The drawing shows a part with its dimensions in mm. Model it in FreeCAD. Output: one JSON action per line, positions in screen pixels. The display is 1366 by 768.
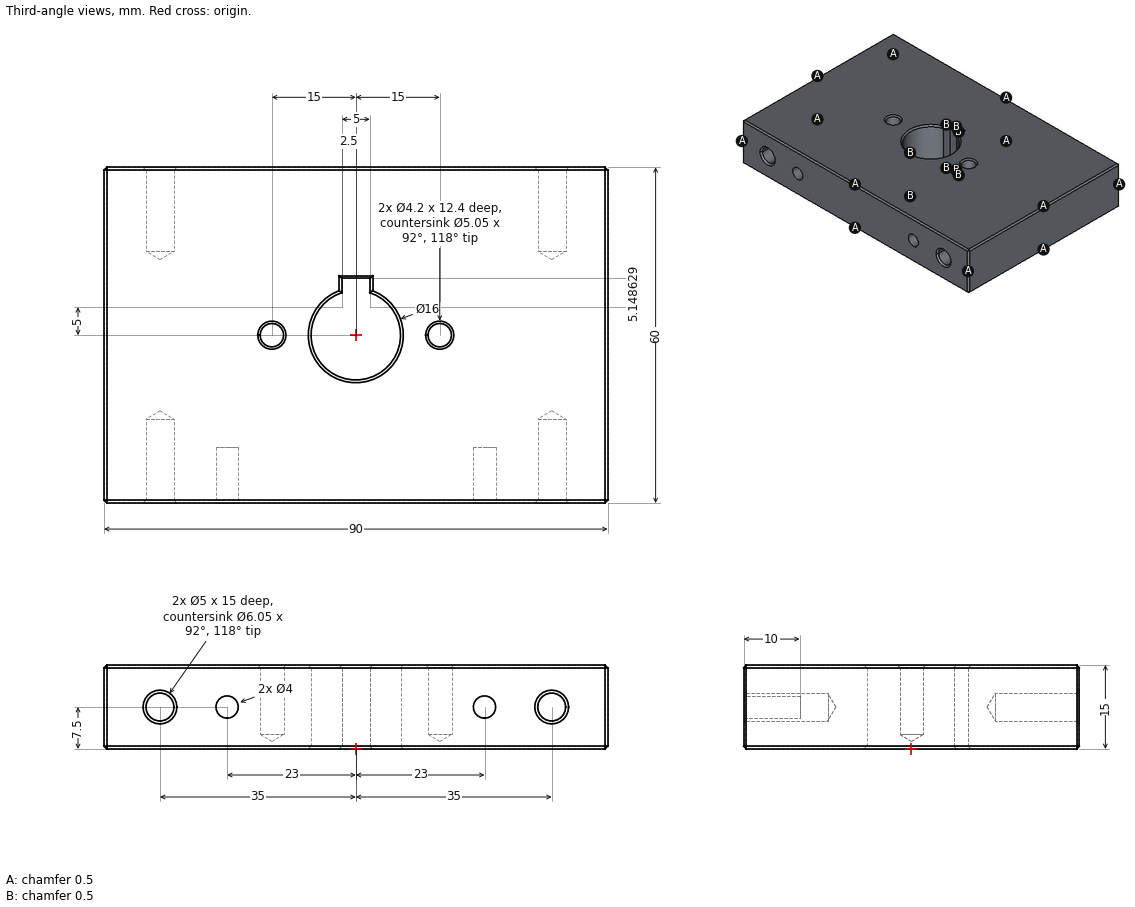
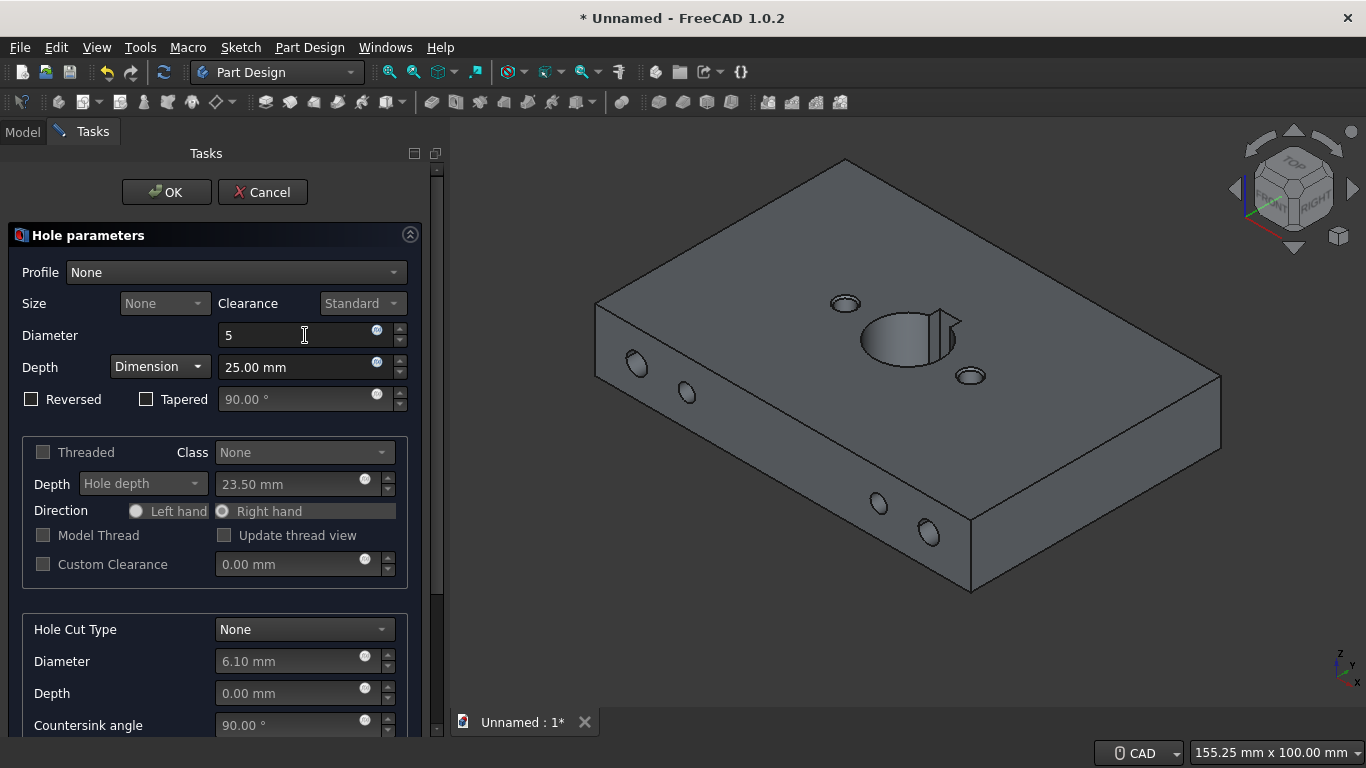
{"action": "triple_click", "coordinate": [305, 367]}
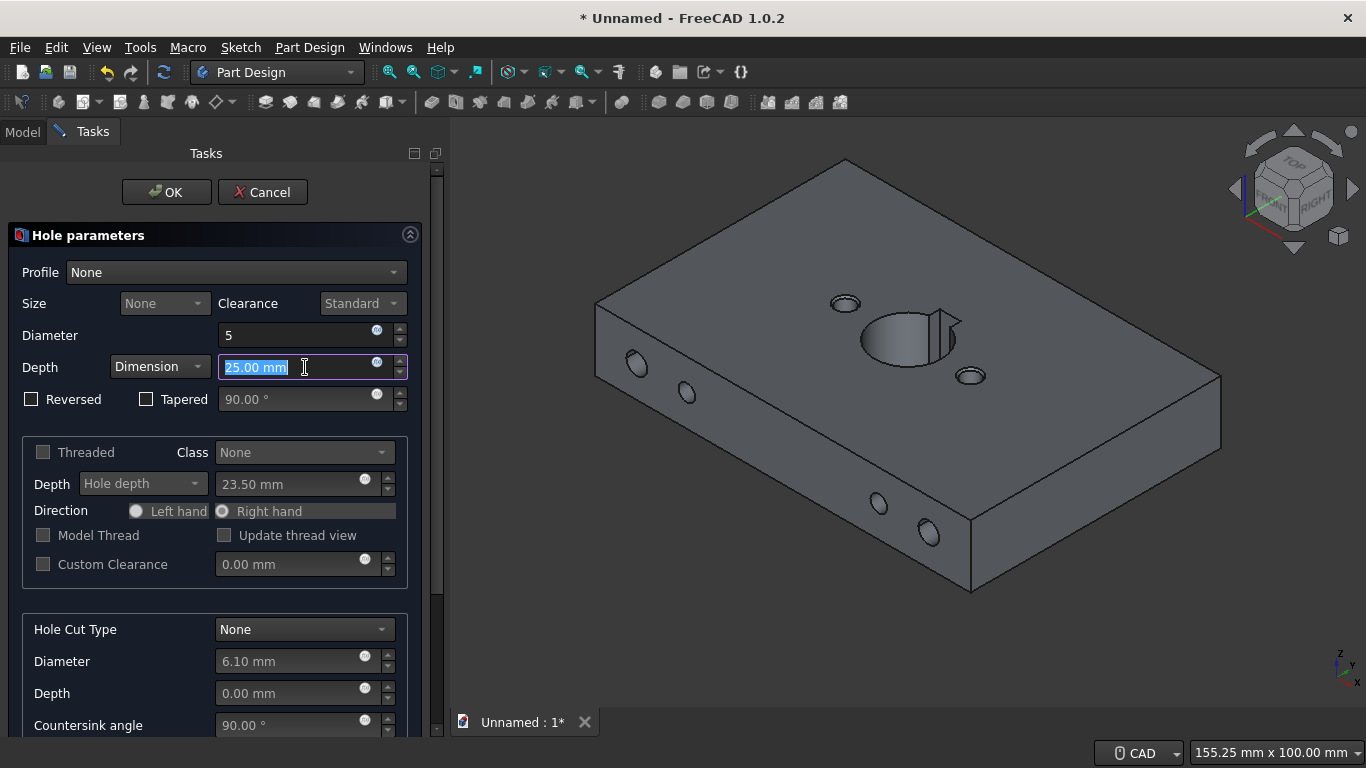
{"action": "type", "text": "15"}
{"action": "key", "text": "Tab"}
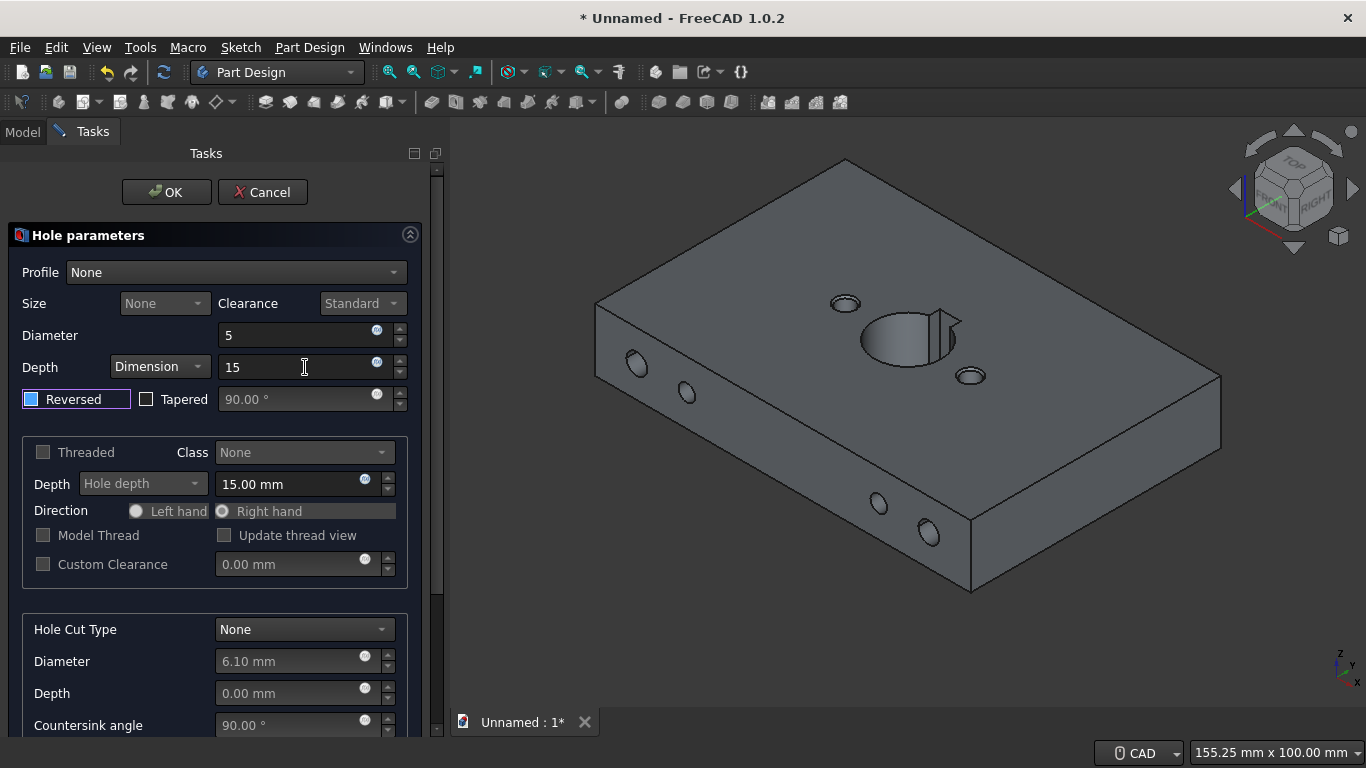
{"action": "left_click", "coordinate": [306, 630]}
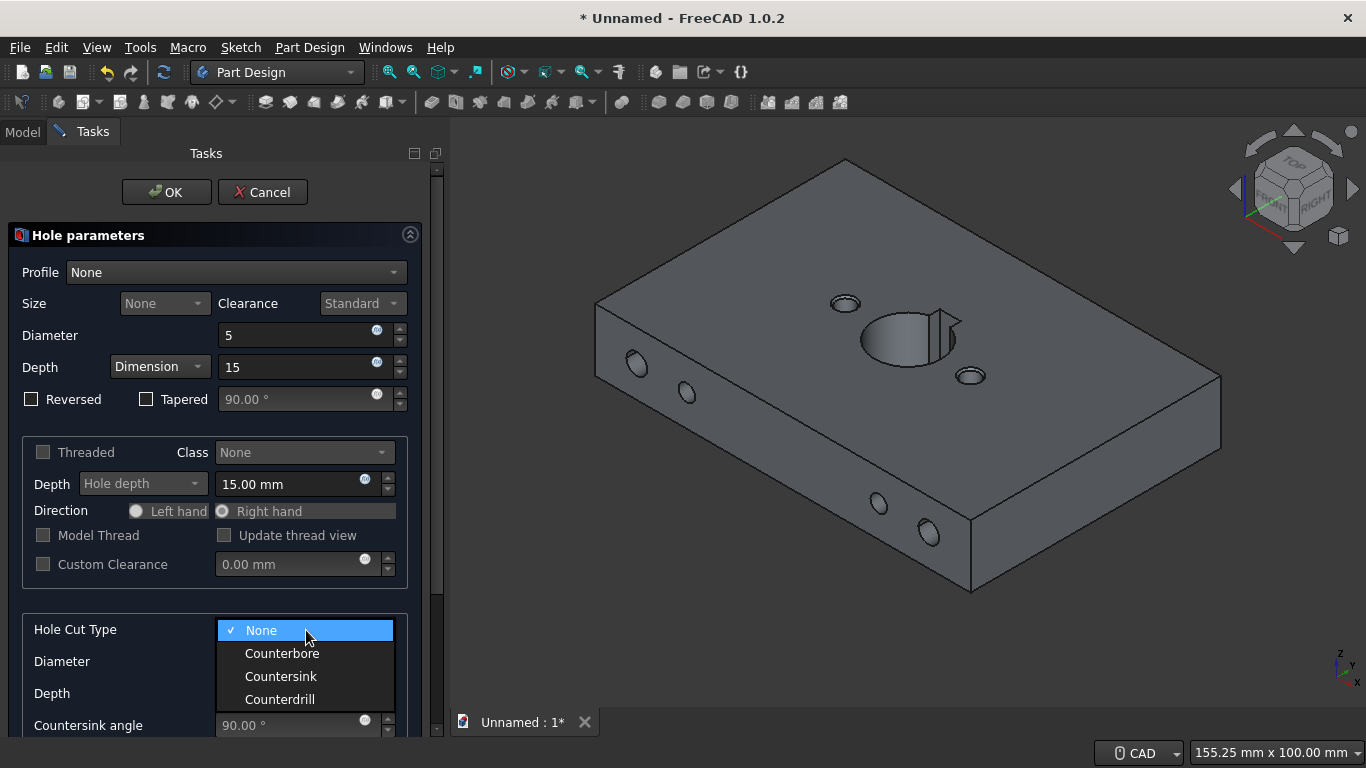
{"action": "left_click", "coordinate": [304, 676]}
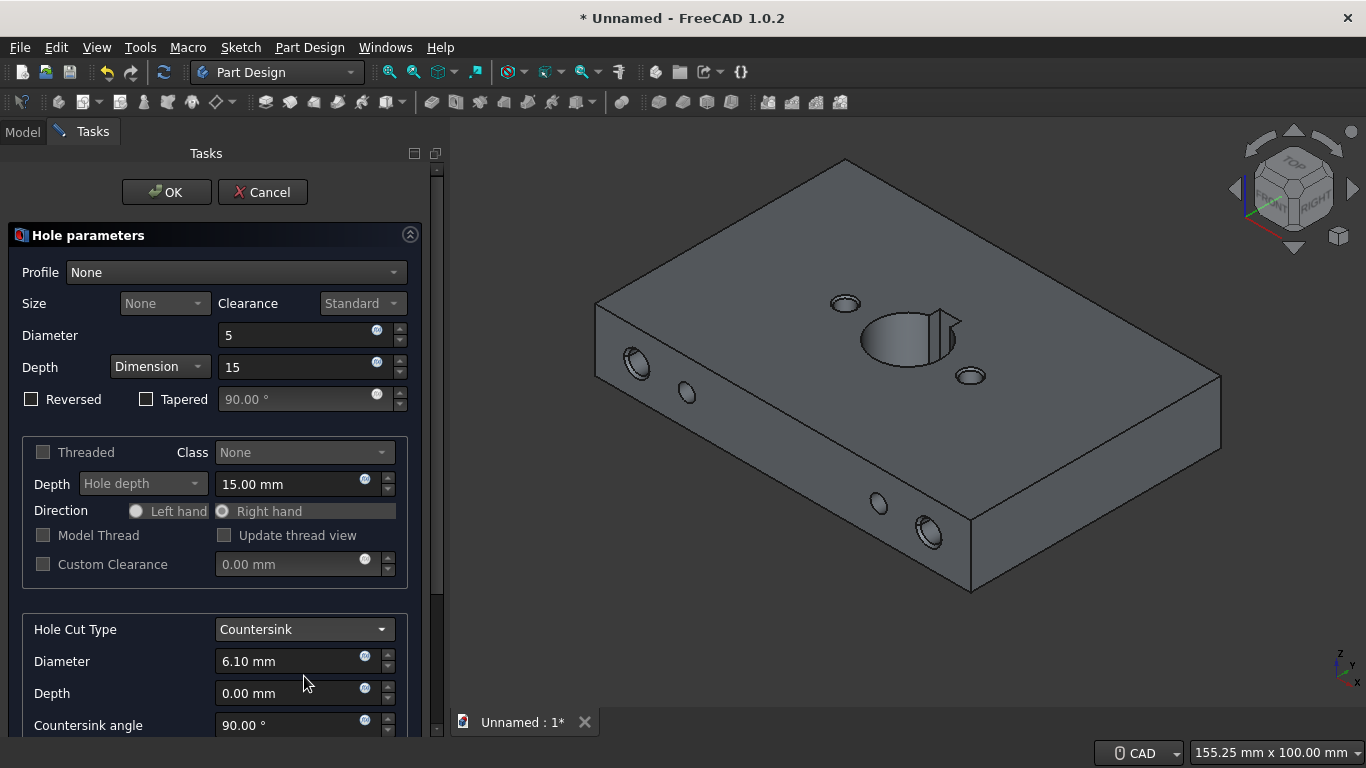
{"action": "scroll", "coordinate": [437, 450], "scroll_direction": "down", "scroll_amount": 2}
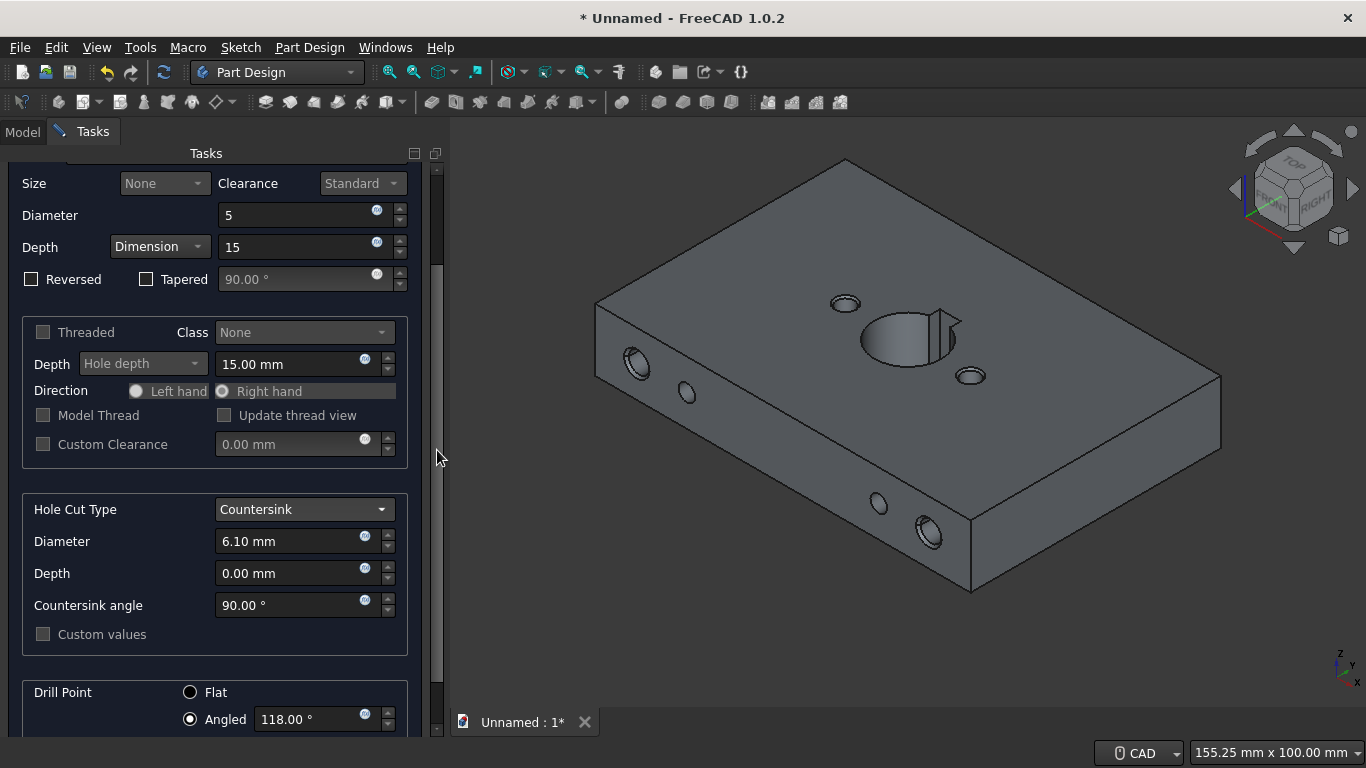
{"action": "triple_click", "coordinate": [298, 605]}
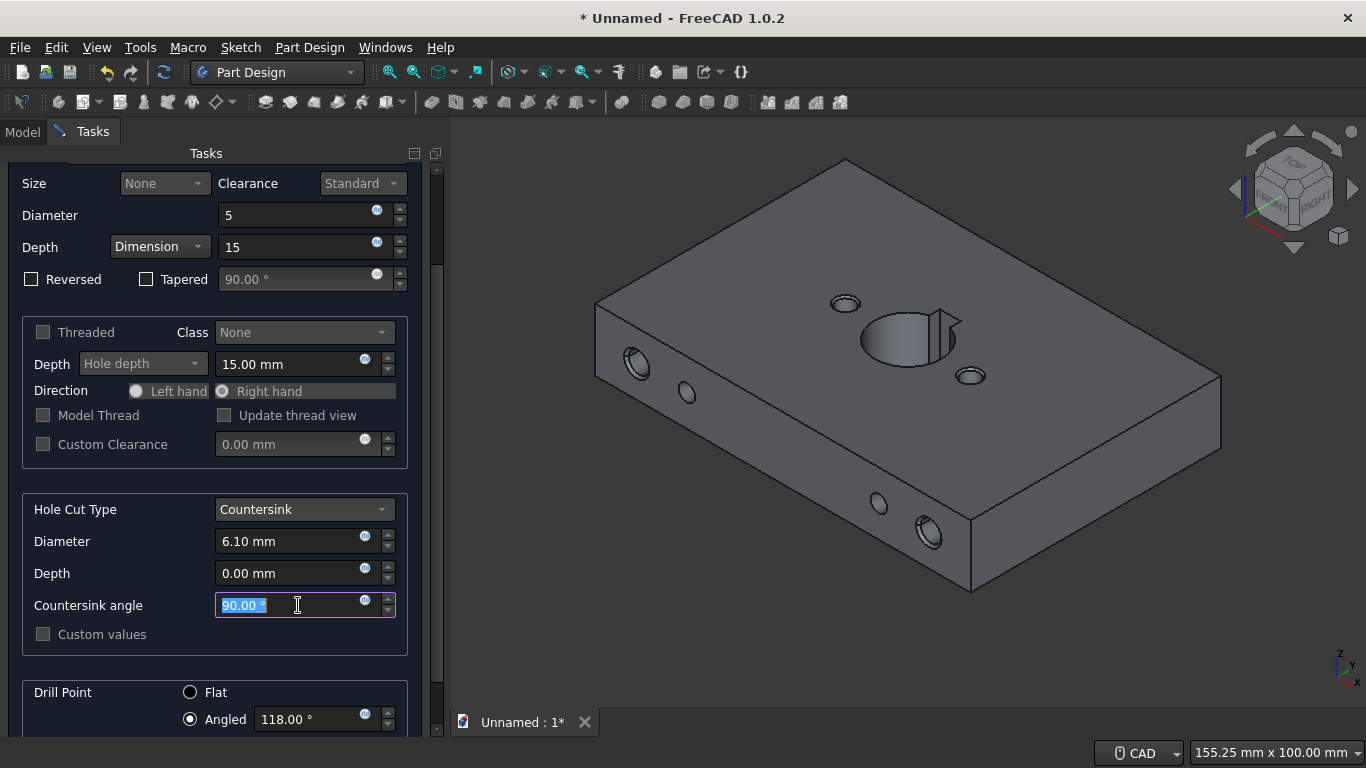
{"action": "type", "text": "92"}
{"action": "key", "text": "Tab"}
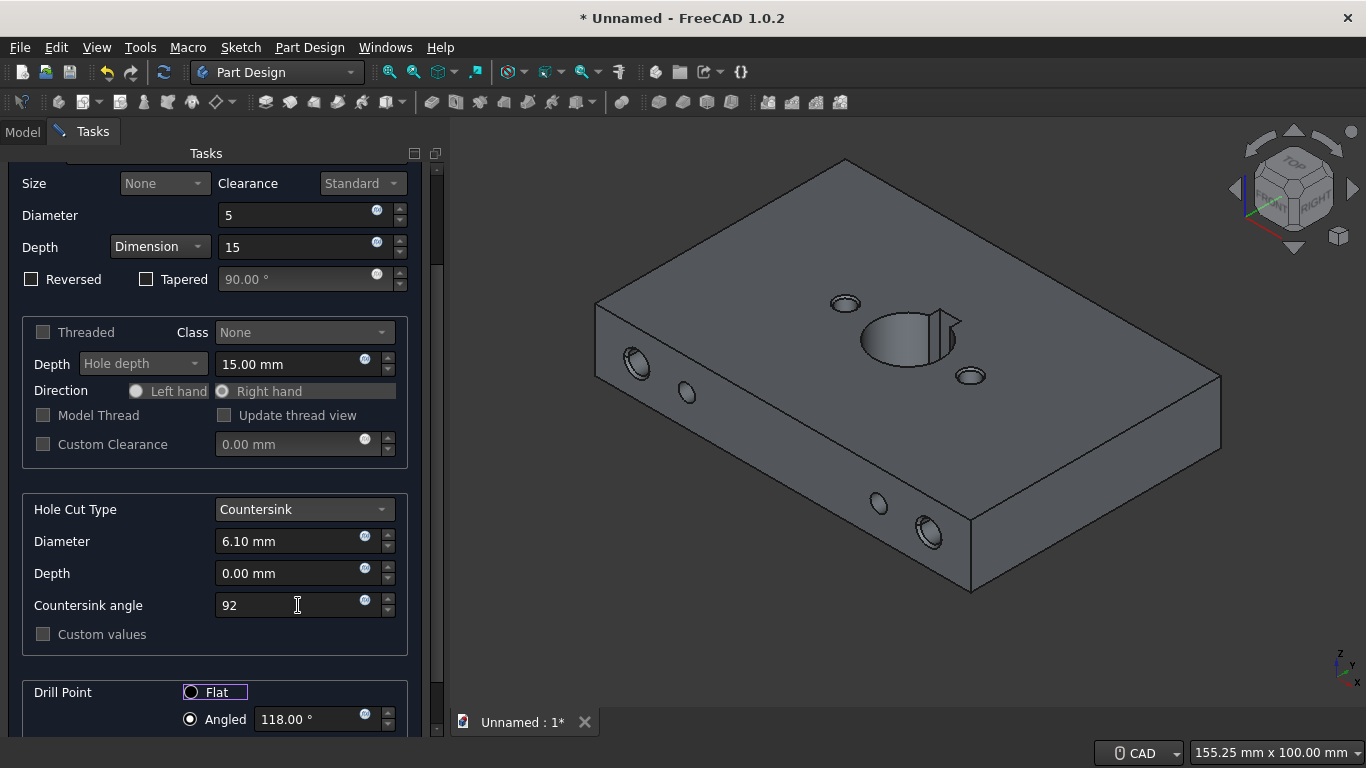
{"action": "triple_click", "coordinate": [298, 541]}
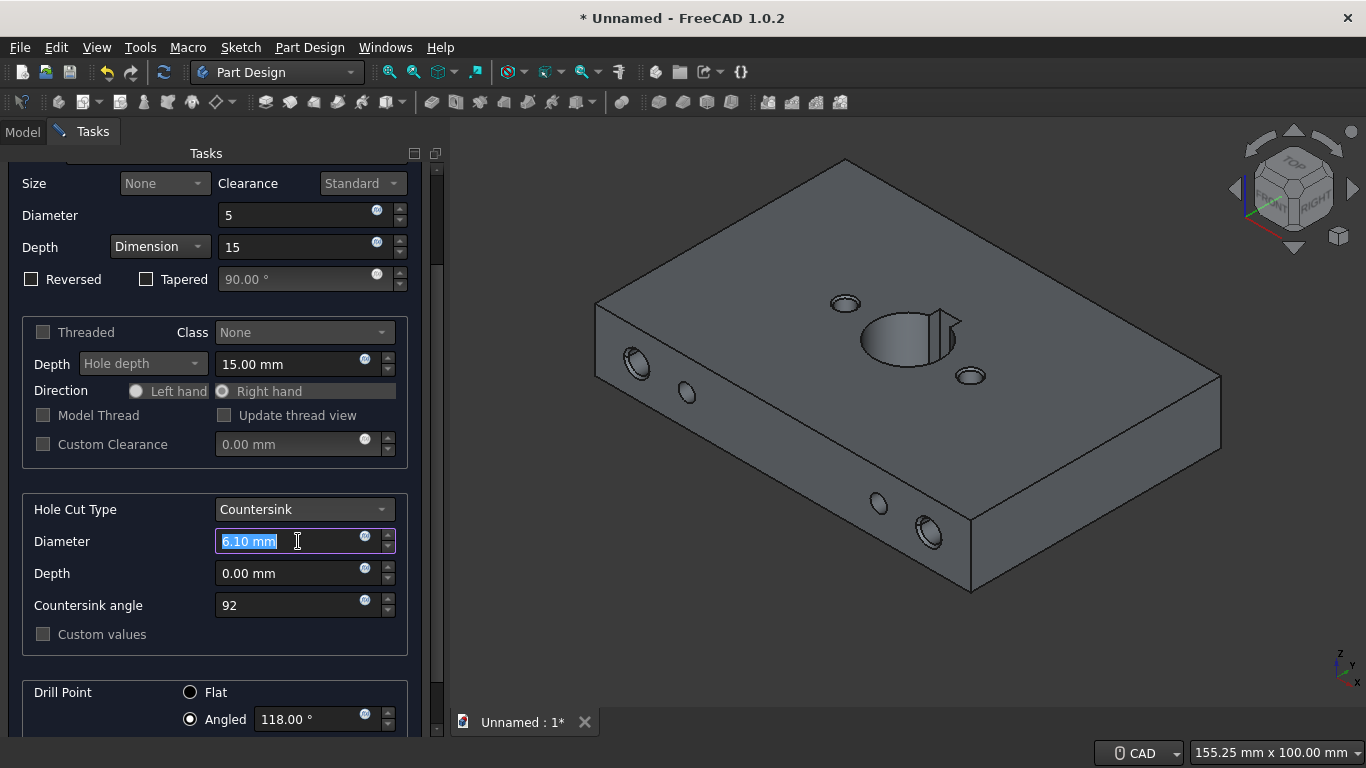
{"action": "type", "text": "6.05"}
{"action": "key", "text": "Tab"}